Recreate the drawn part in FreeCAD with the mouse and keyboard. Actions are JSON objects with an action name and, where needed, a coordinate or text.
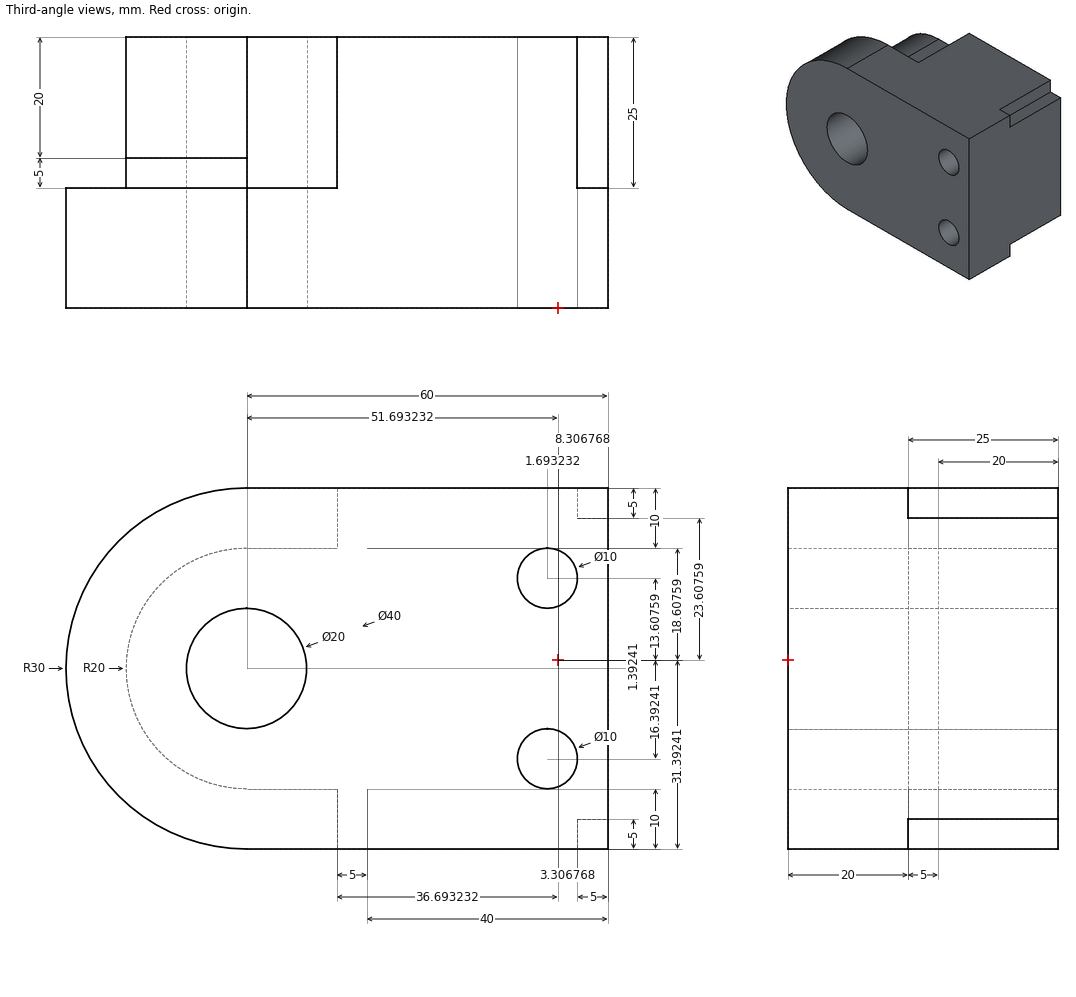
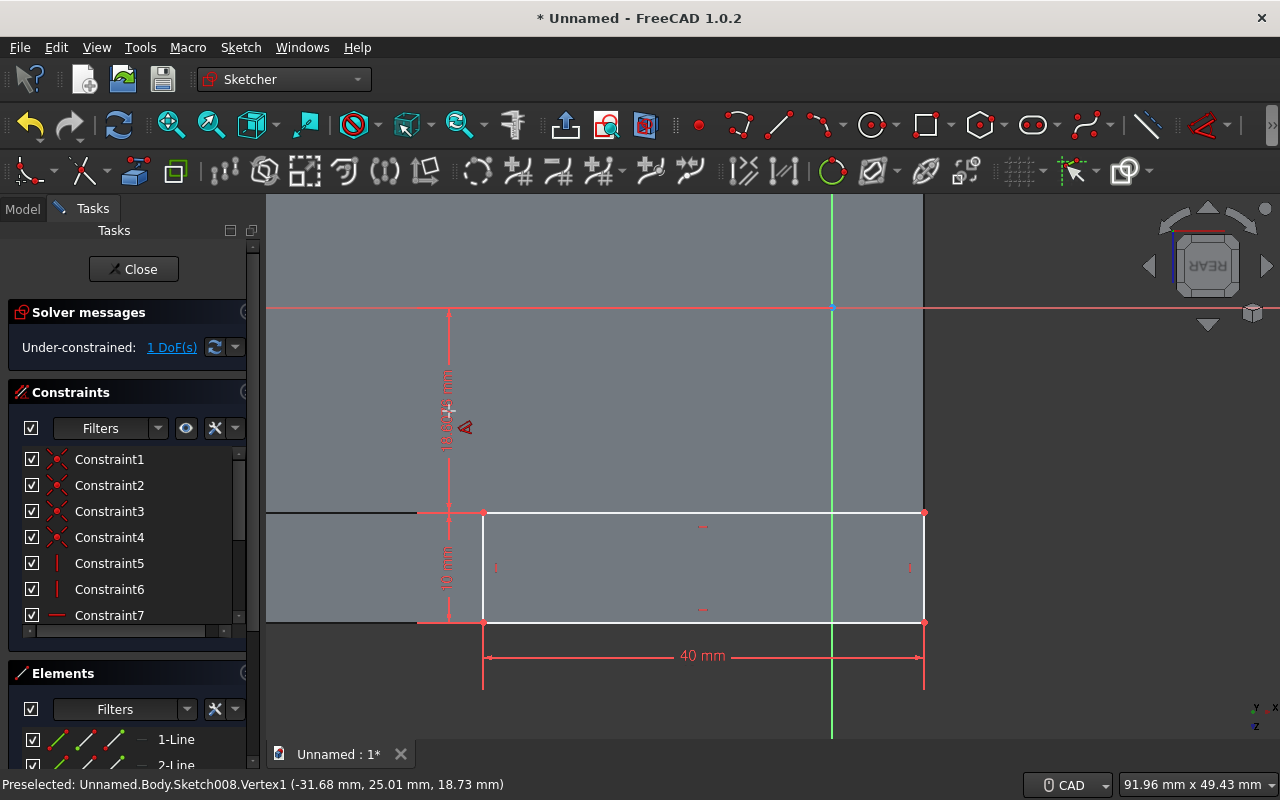
{"action": "left_click", "coordinate": [924, 623]}
{"action": "left_click", "coordinate": [878, 657]}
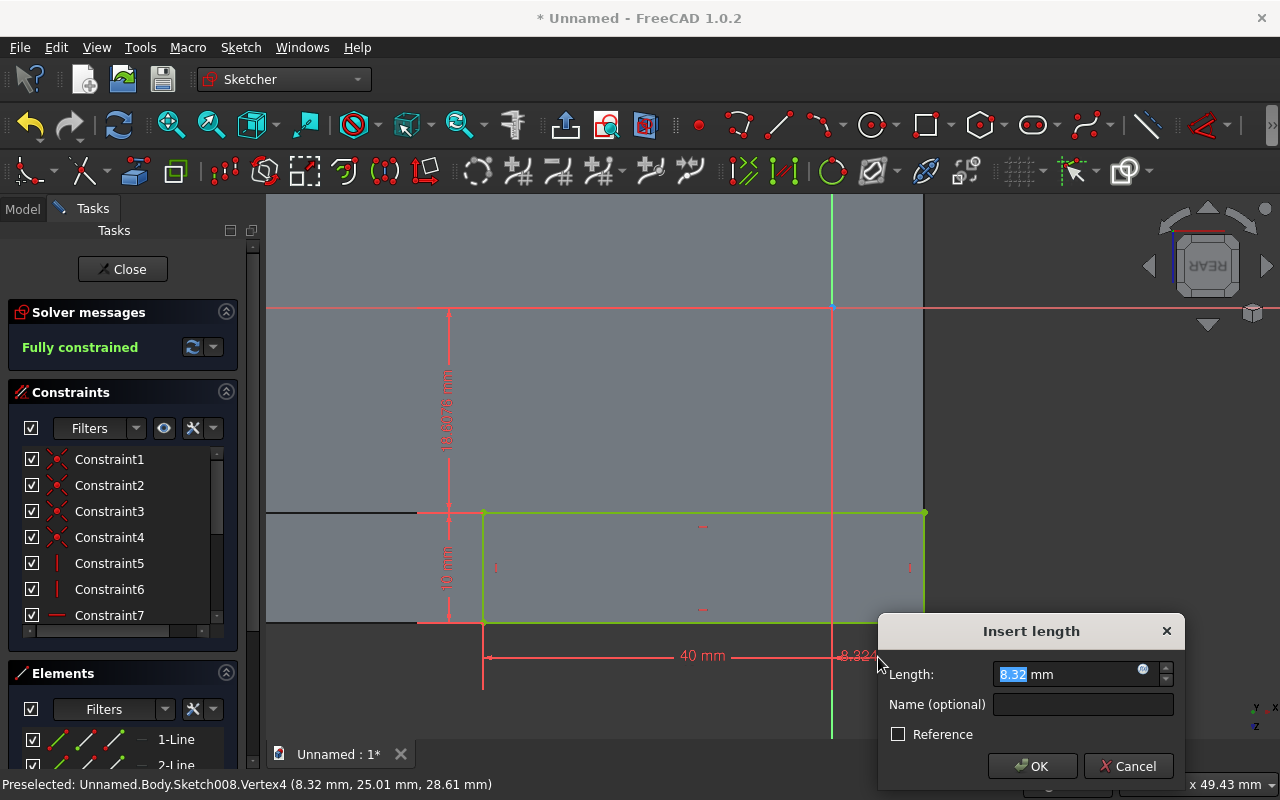
{"action": "type", "text": "8.306768"}
{"action": "key", "text": "Return"}
{"action": "key", "text": "Escape"}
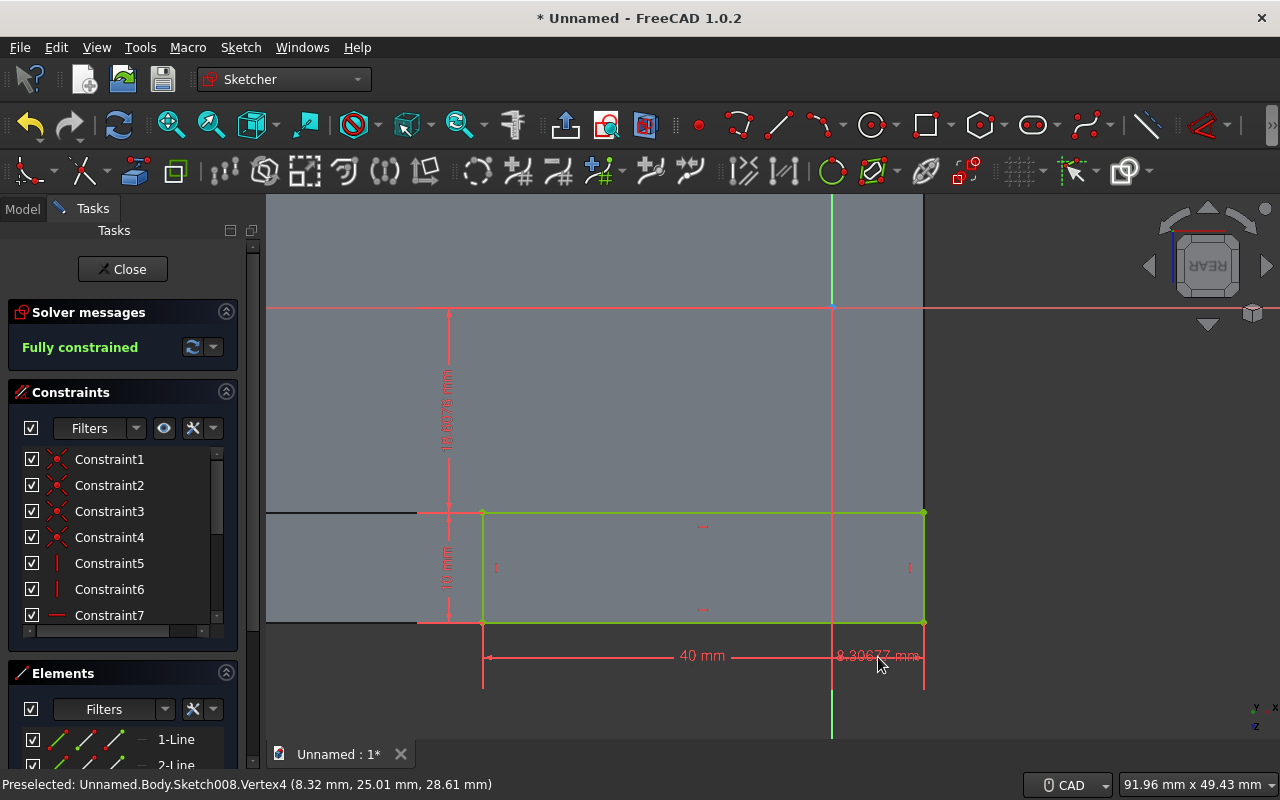
{"action": "left_click", "coordinate": [123, 269]}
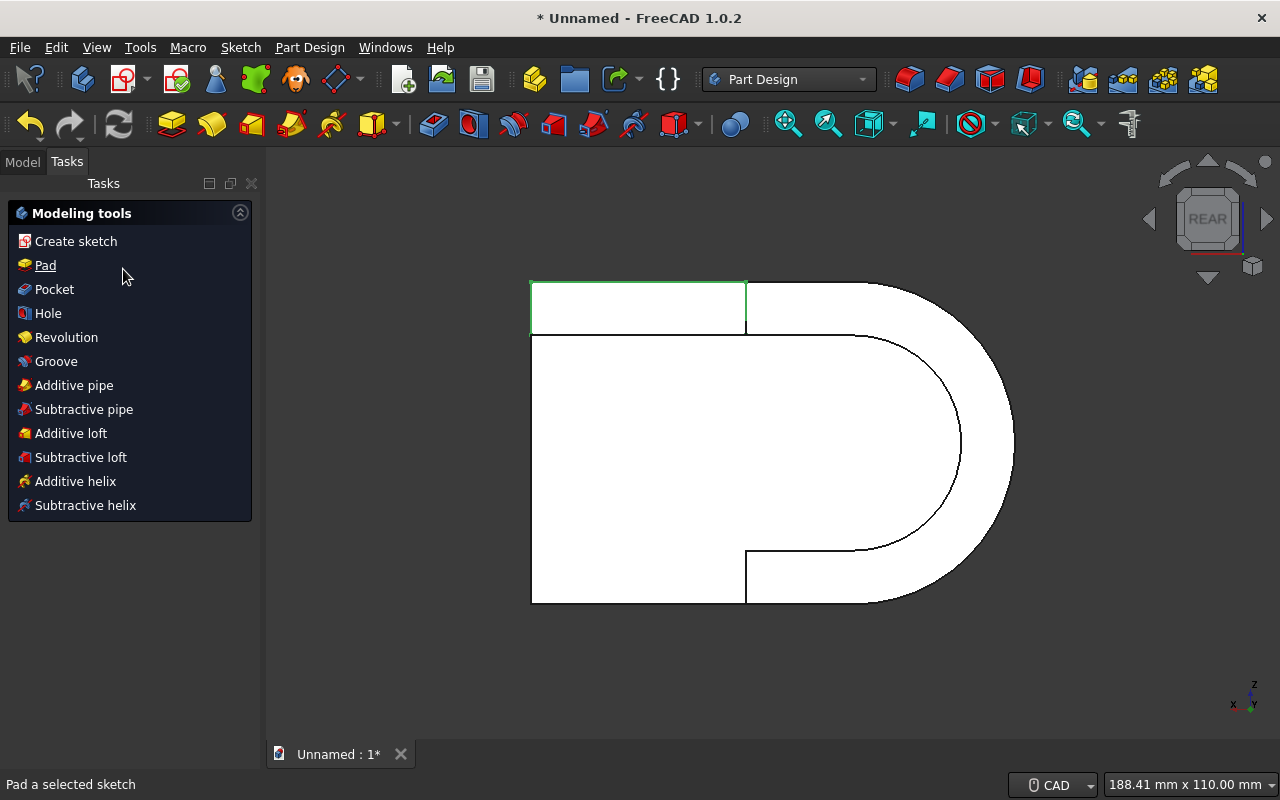
{"action": "left_click", "coordinate": [172, 124]}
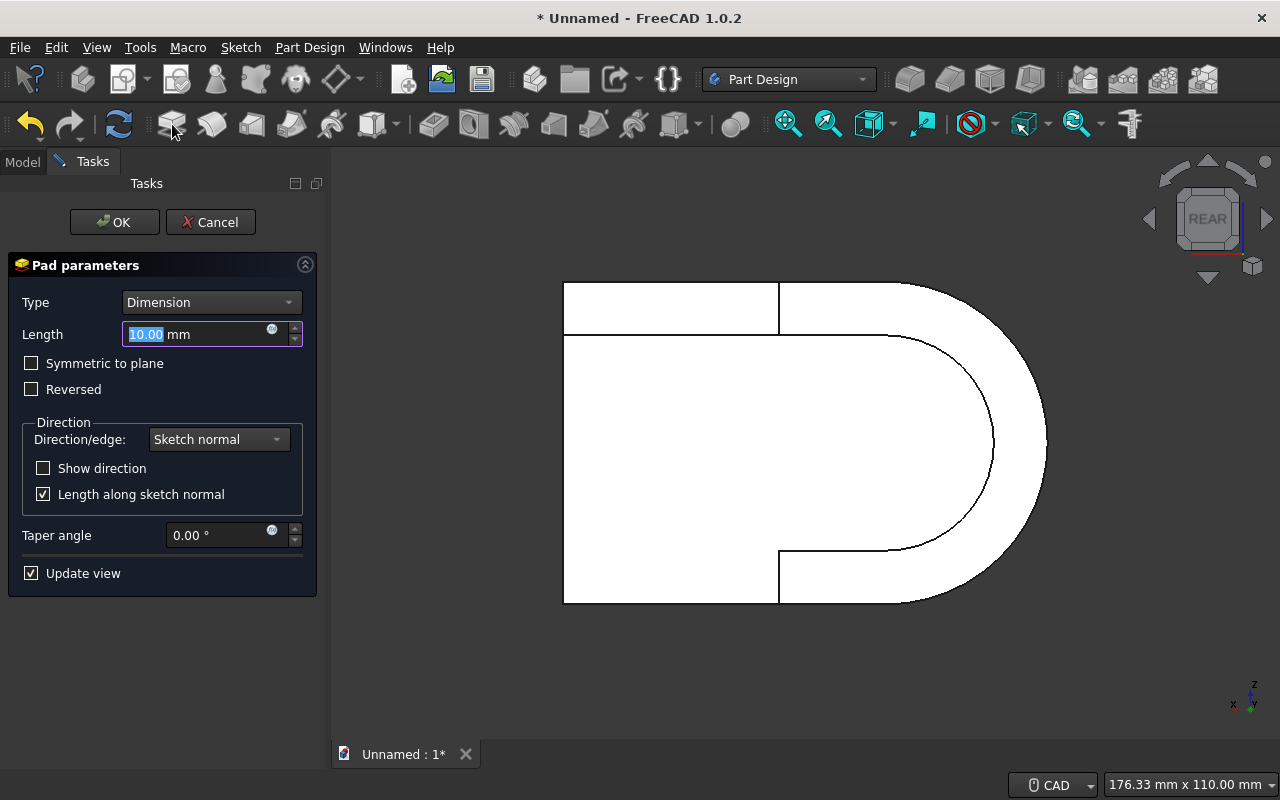
{"action": "type", "text": "20"}
{"action": "key", "text": "Tab"}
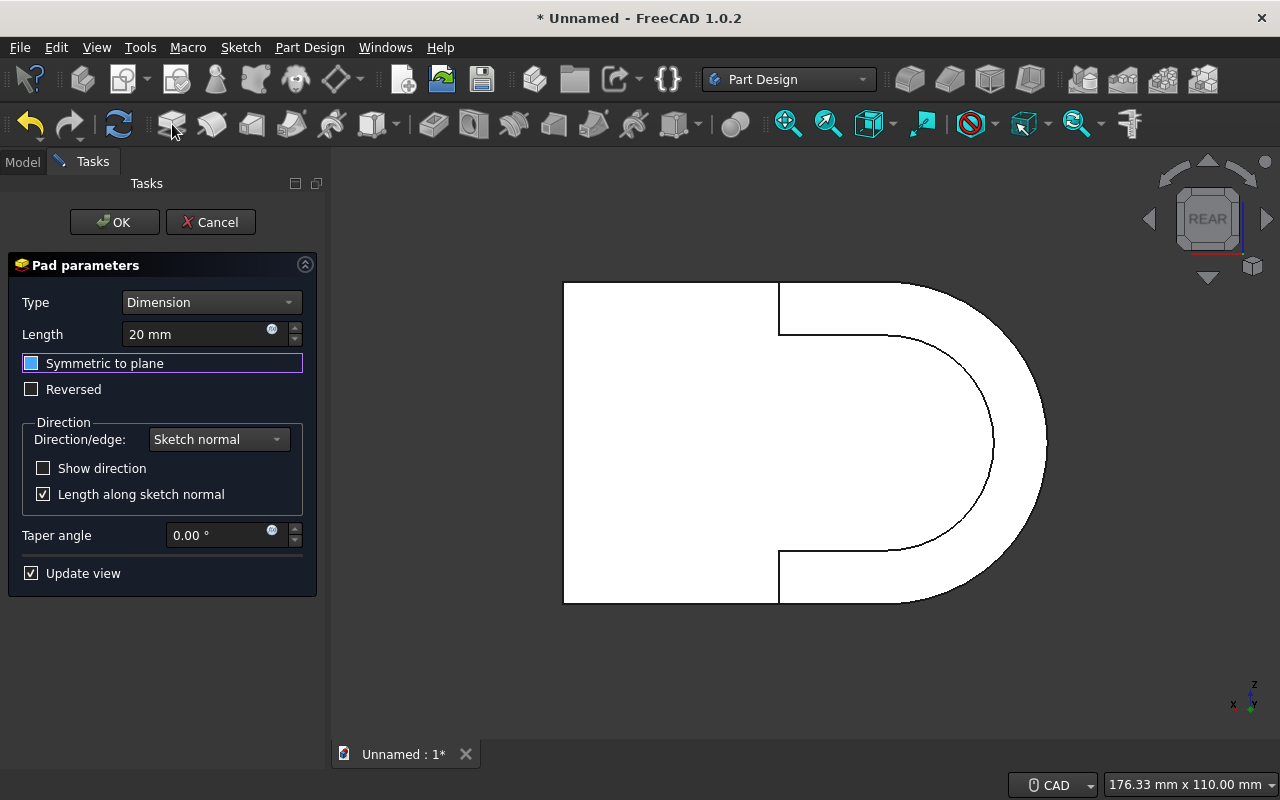
{"action": "left_click", "coordinate": [115, 222]}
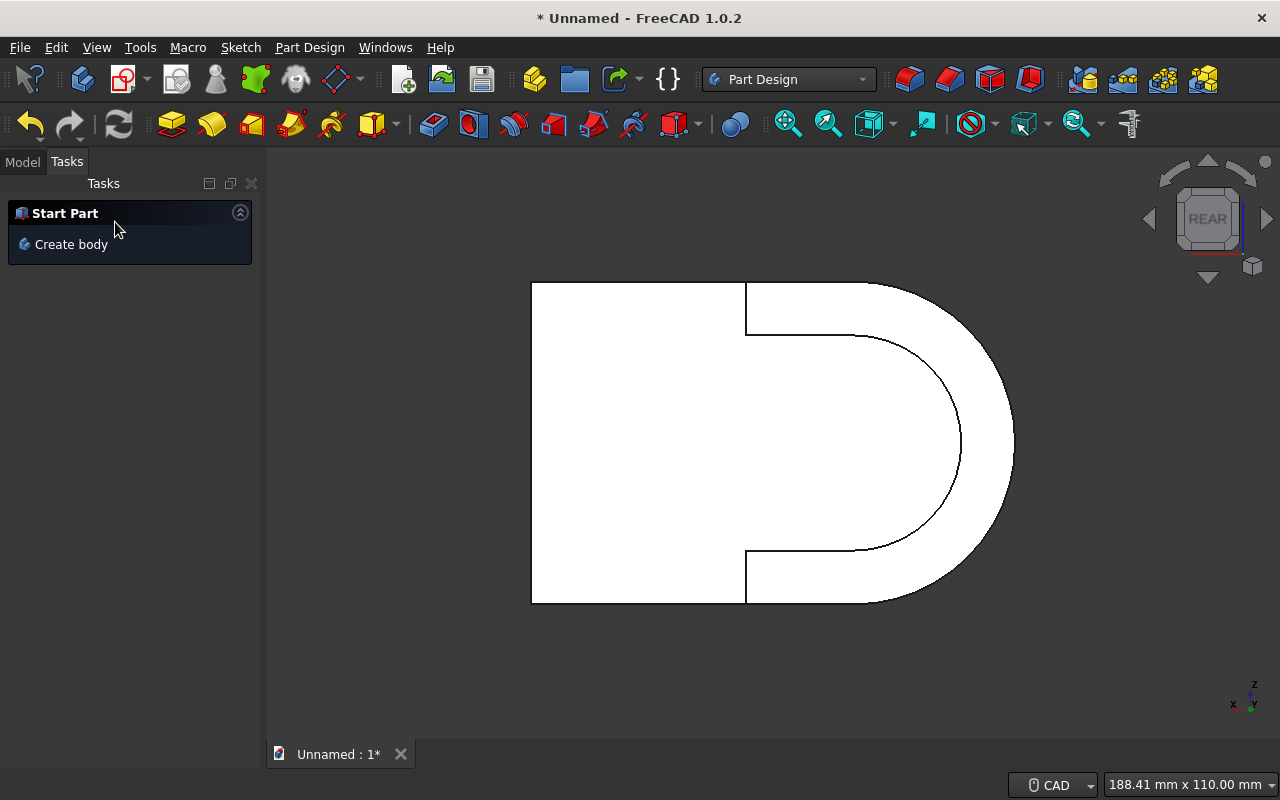
{"action": "left_click", "coordinate": [685, 442]}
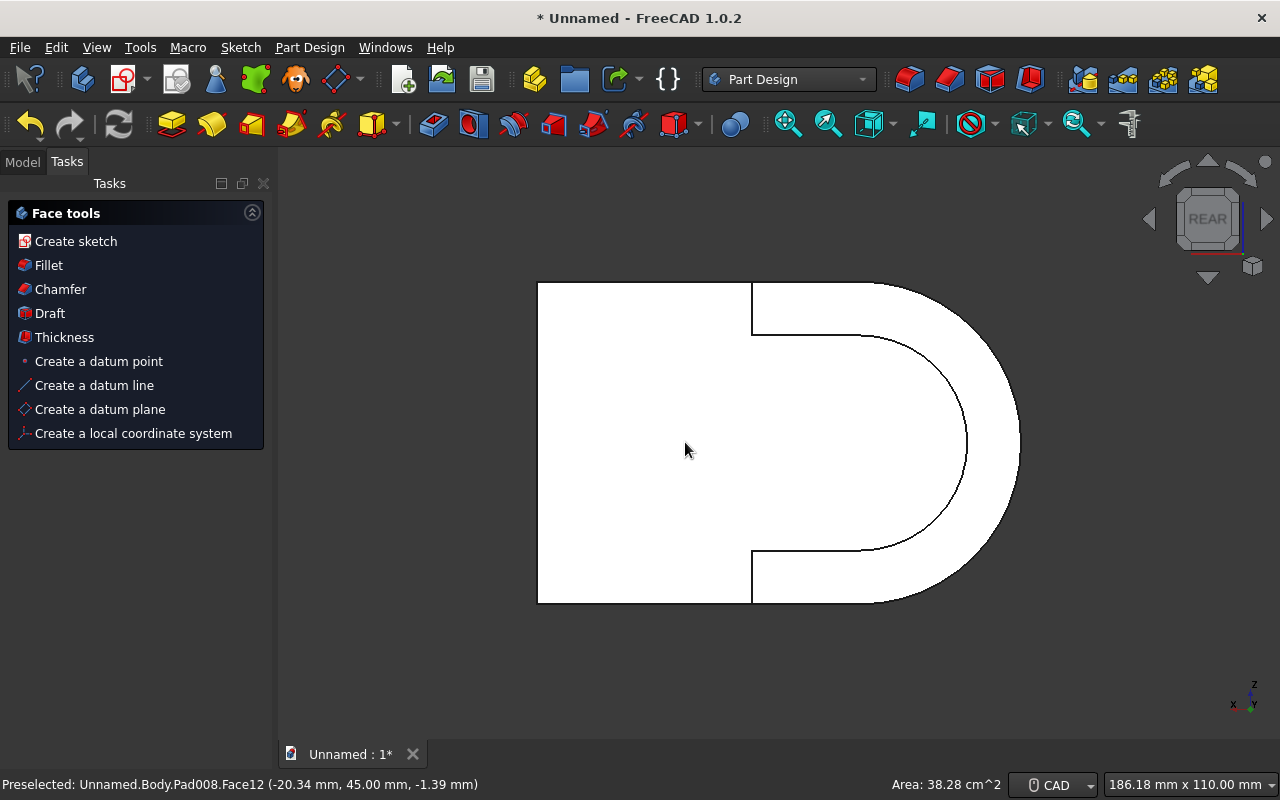
{"action": "left_click", "coordinate": [124, 80]}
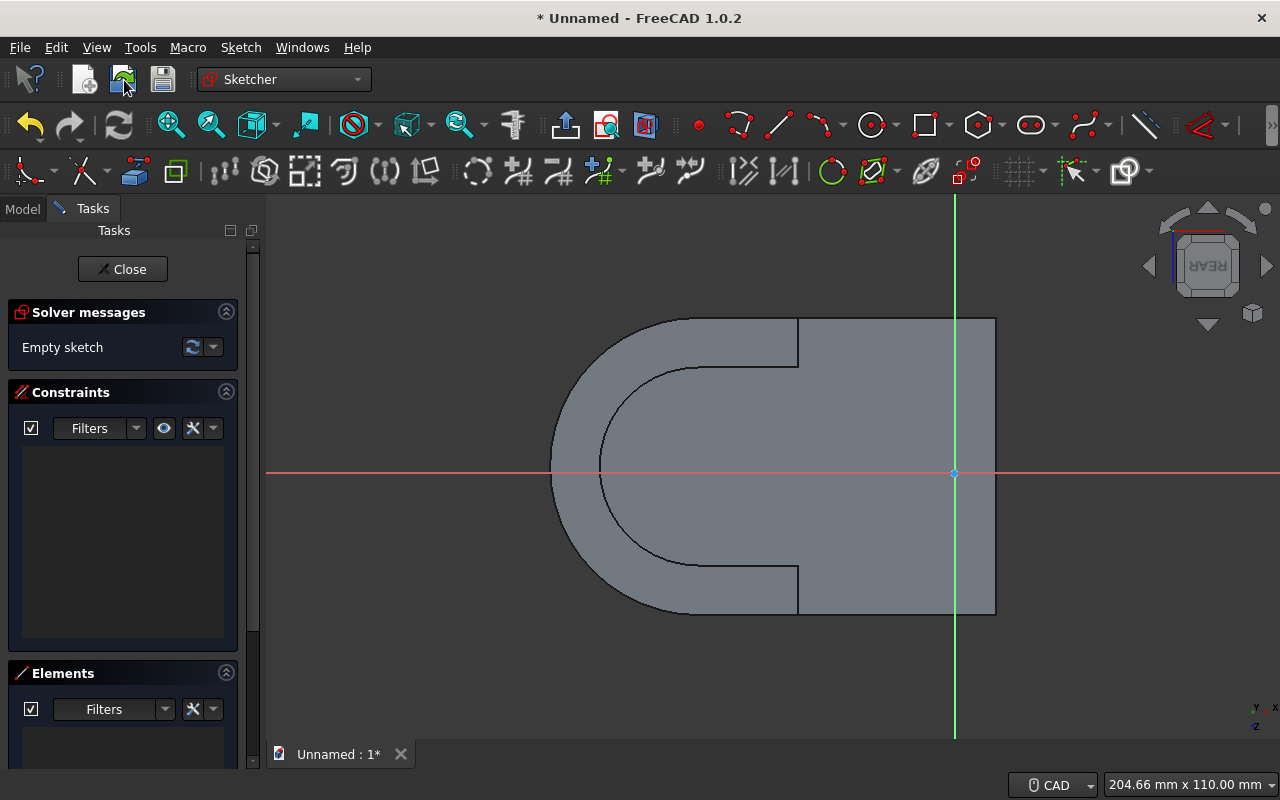
{"action": "scroll", "coordinate": [696, 466], "scroll_direction": "up", "scroll_amount": 6}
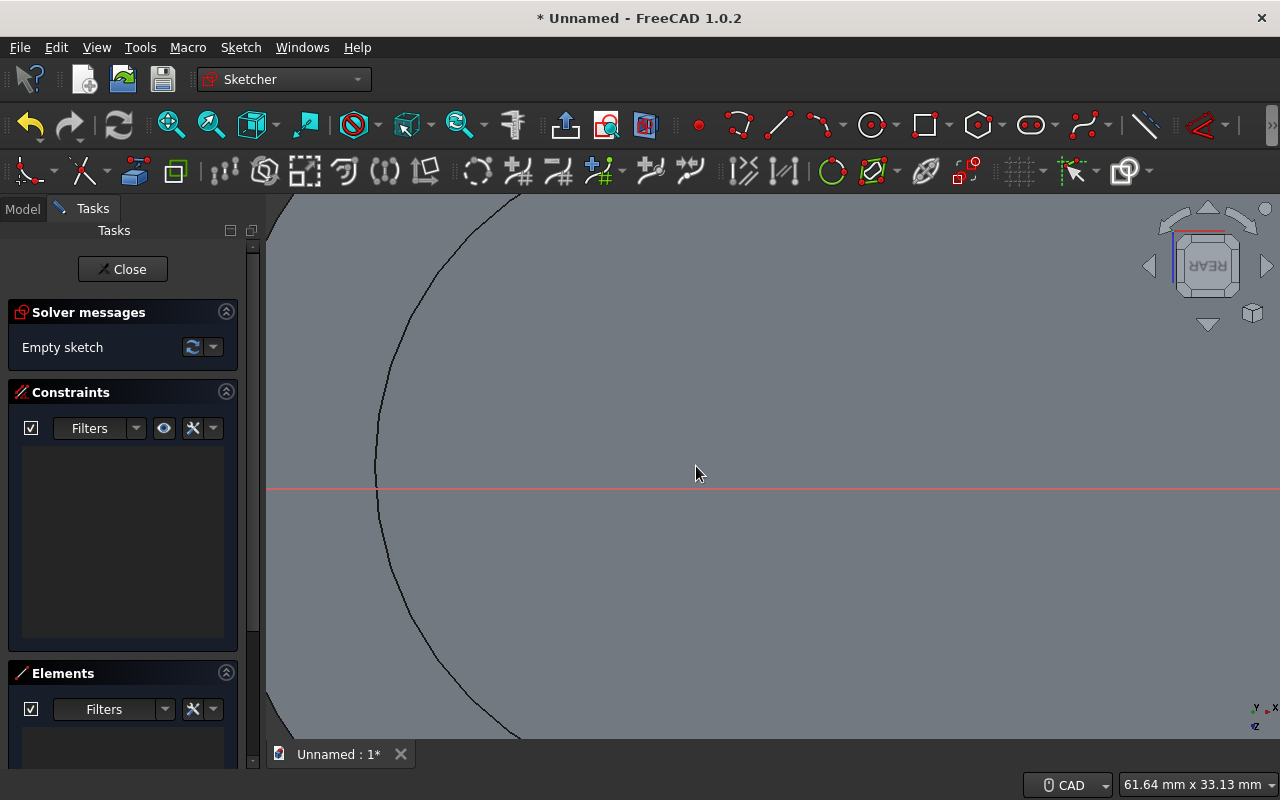
{"action": "left_click", "coordinate": [872, 126]}